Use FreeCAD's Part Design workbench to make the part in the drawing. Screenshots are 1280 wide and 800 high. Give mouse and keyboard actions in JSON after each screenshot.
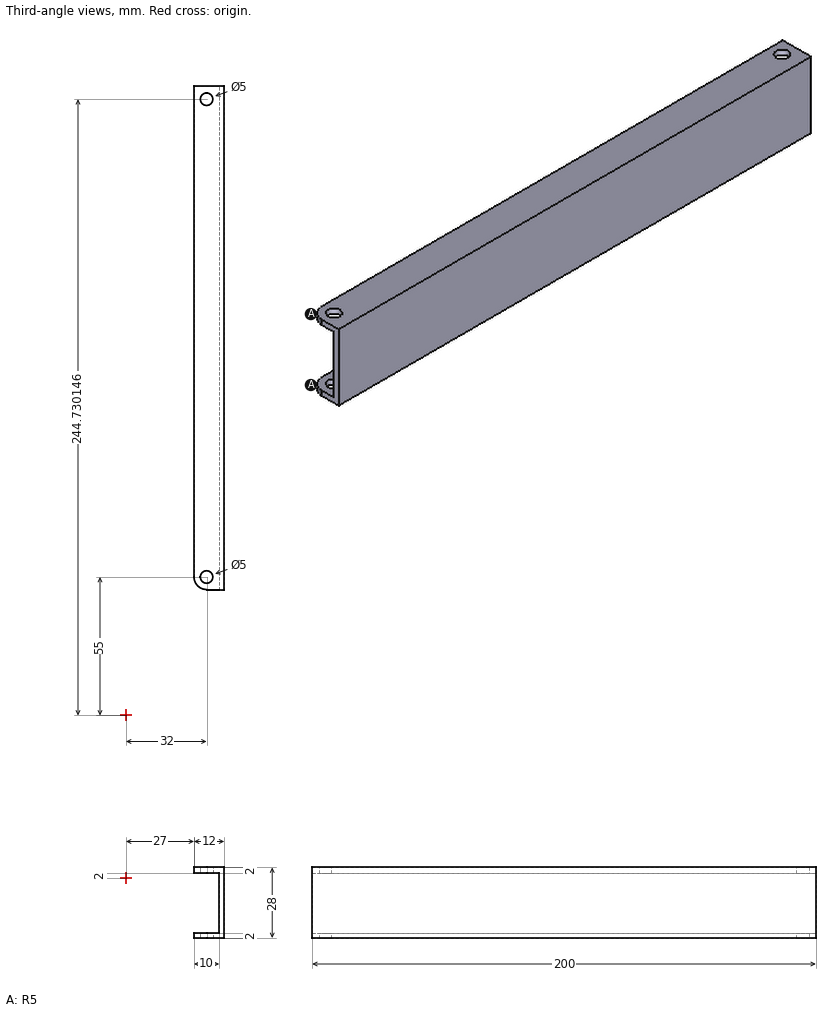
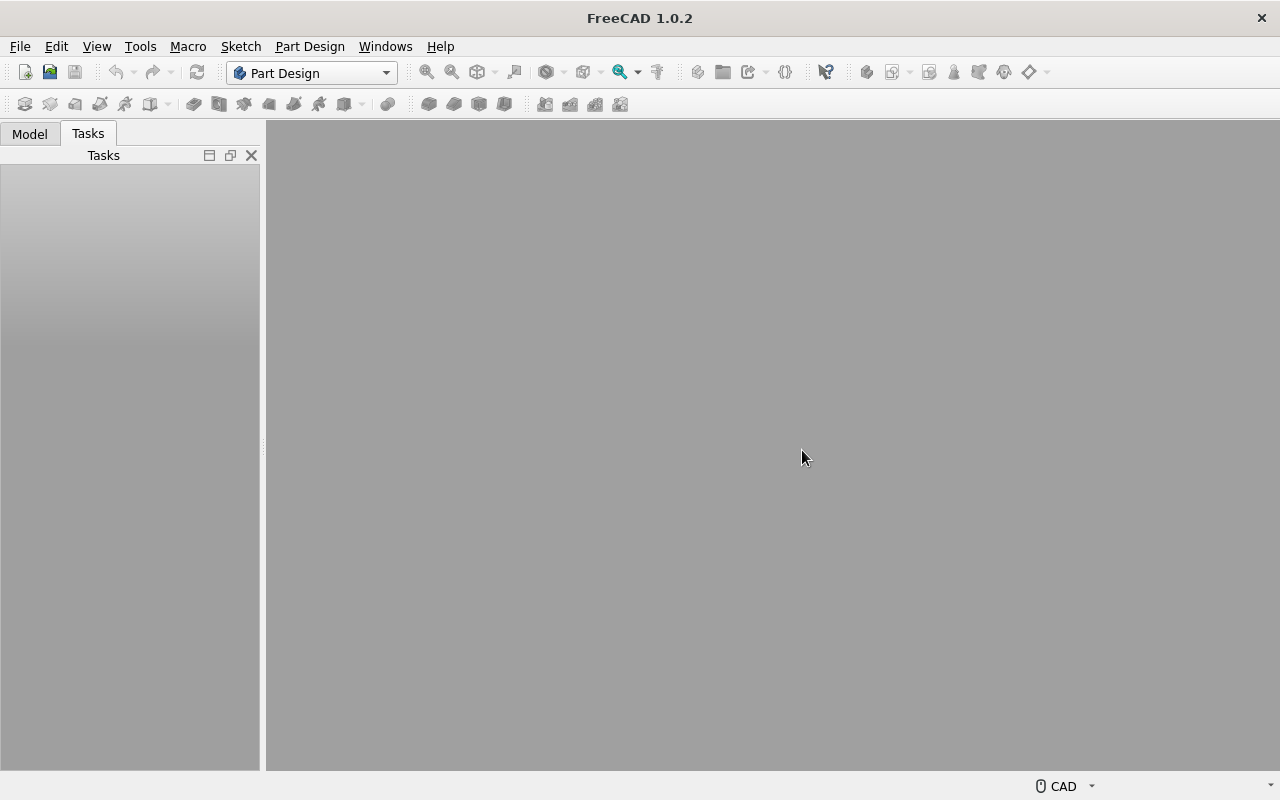
{"action": "left_click", "coordinate": [25, 72]}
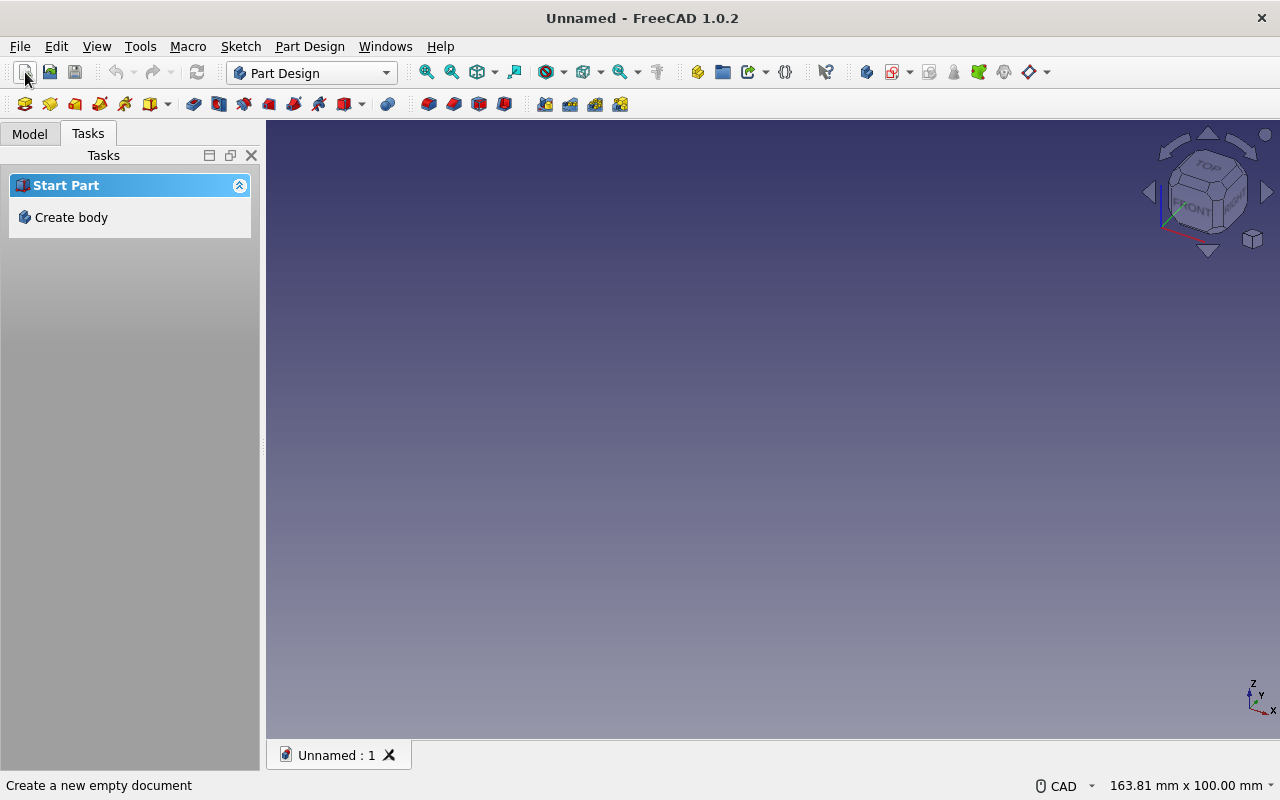
{"action": "left_click", "coordinate": [867, 72]}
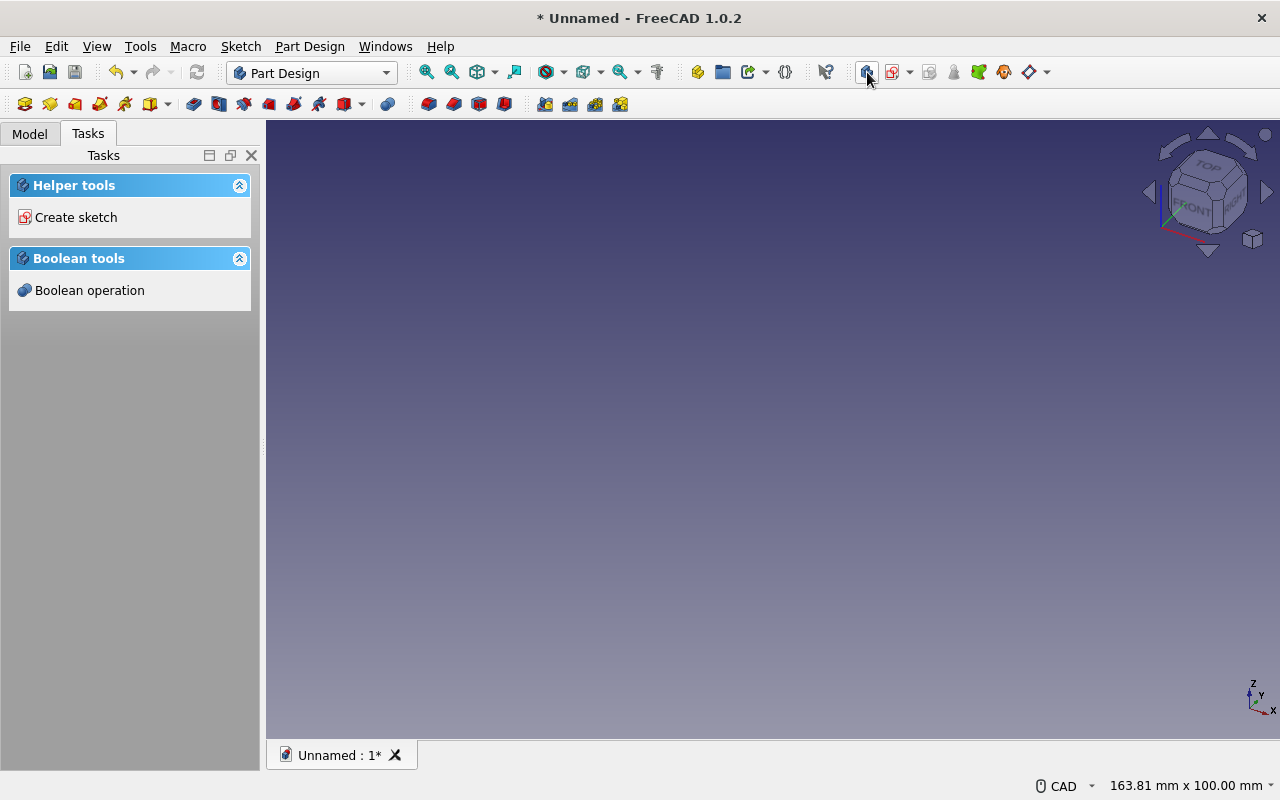
{"action": "left_click", "coordinate": [30, 134]}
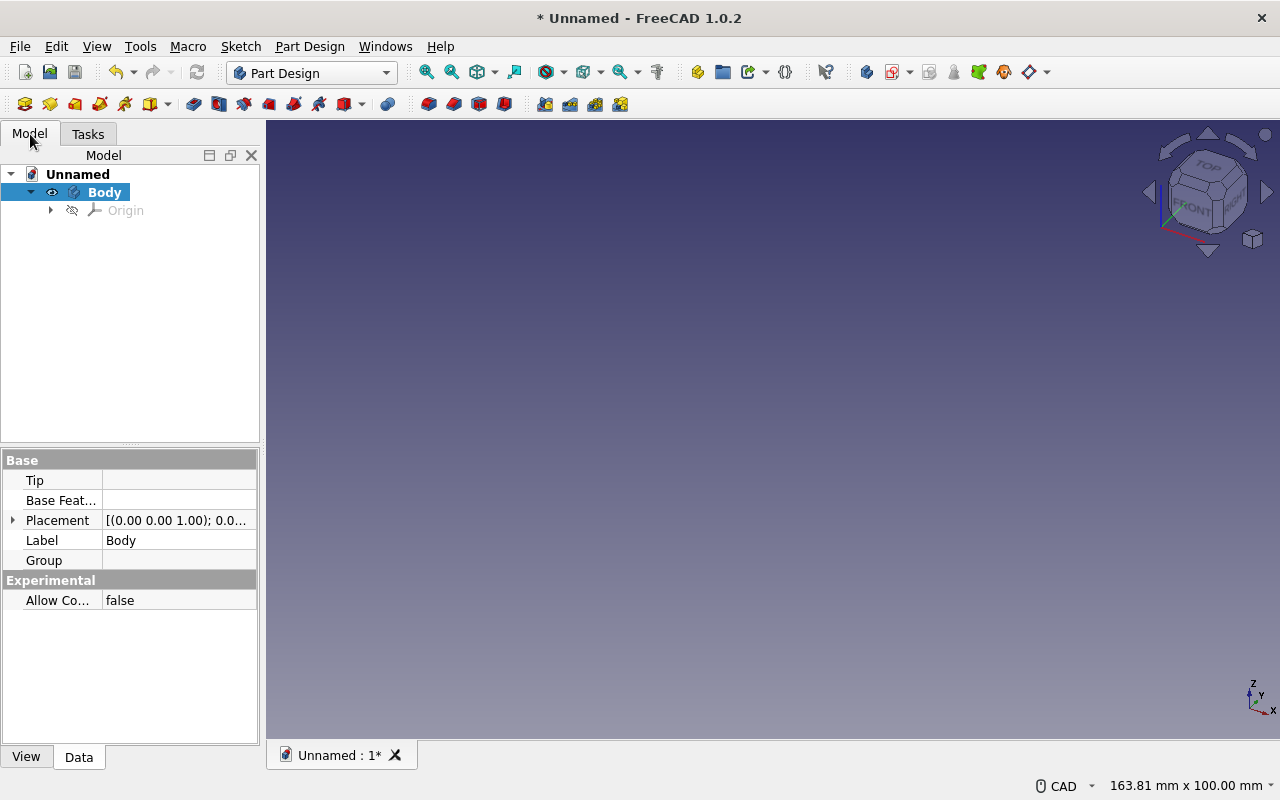
{"action": "left_click", "coordinate": [51, 210]}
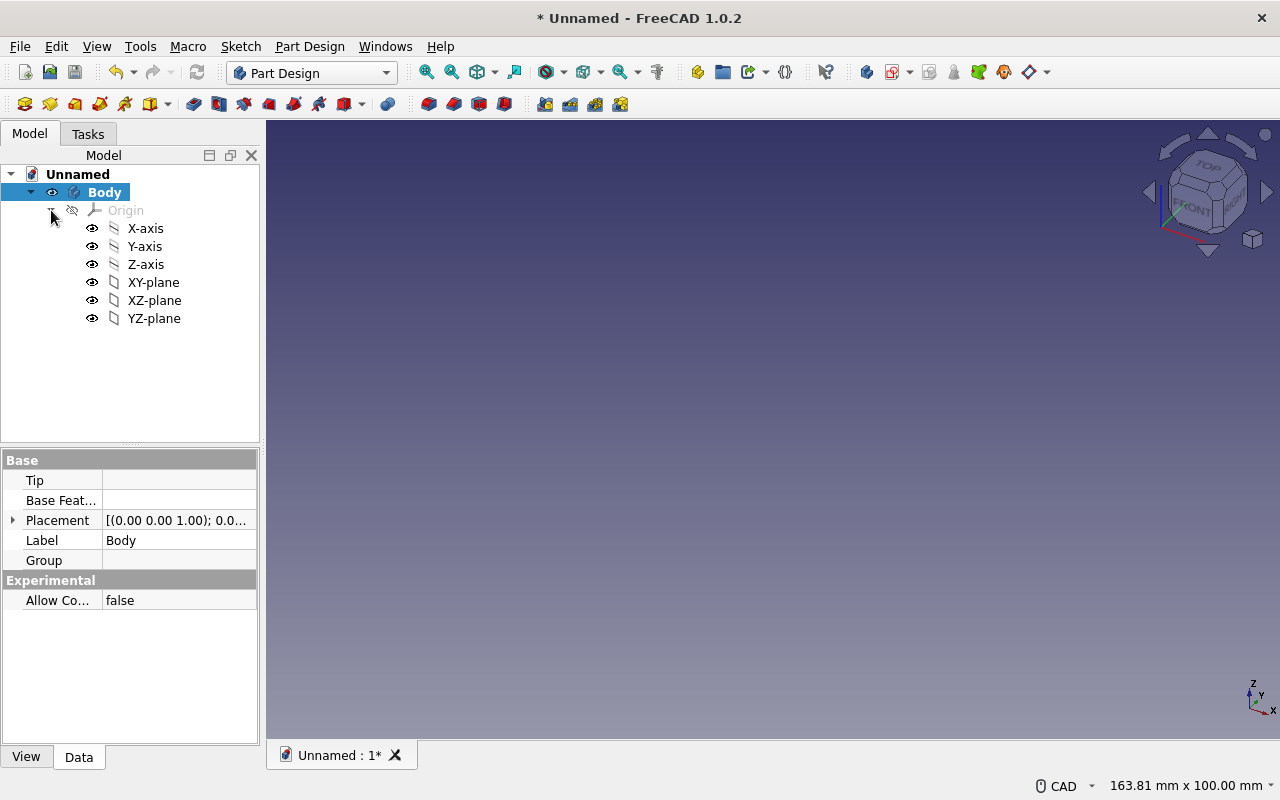
{"action": "left_click", "coordinate": [137, 300]}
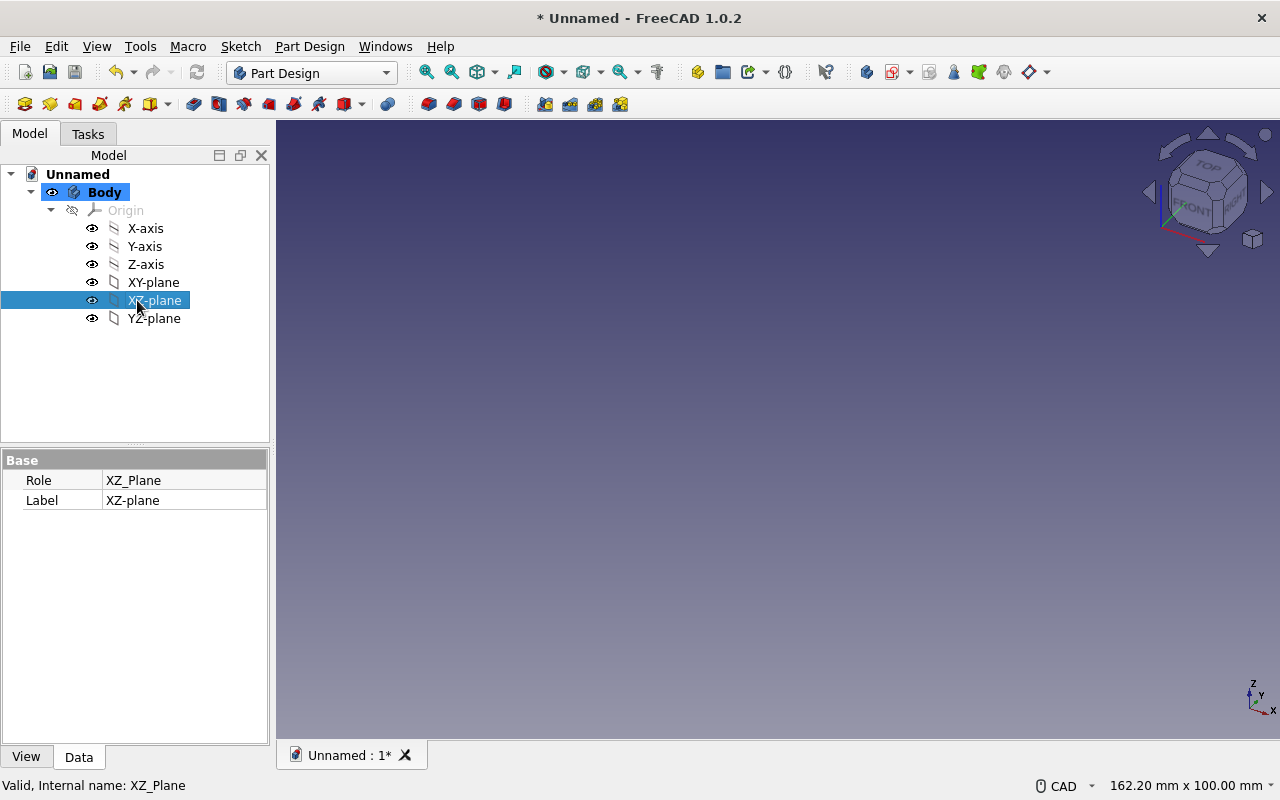
{"action": "left_click", "coordinate": [1028, 72]}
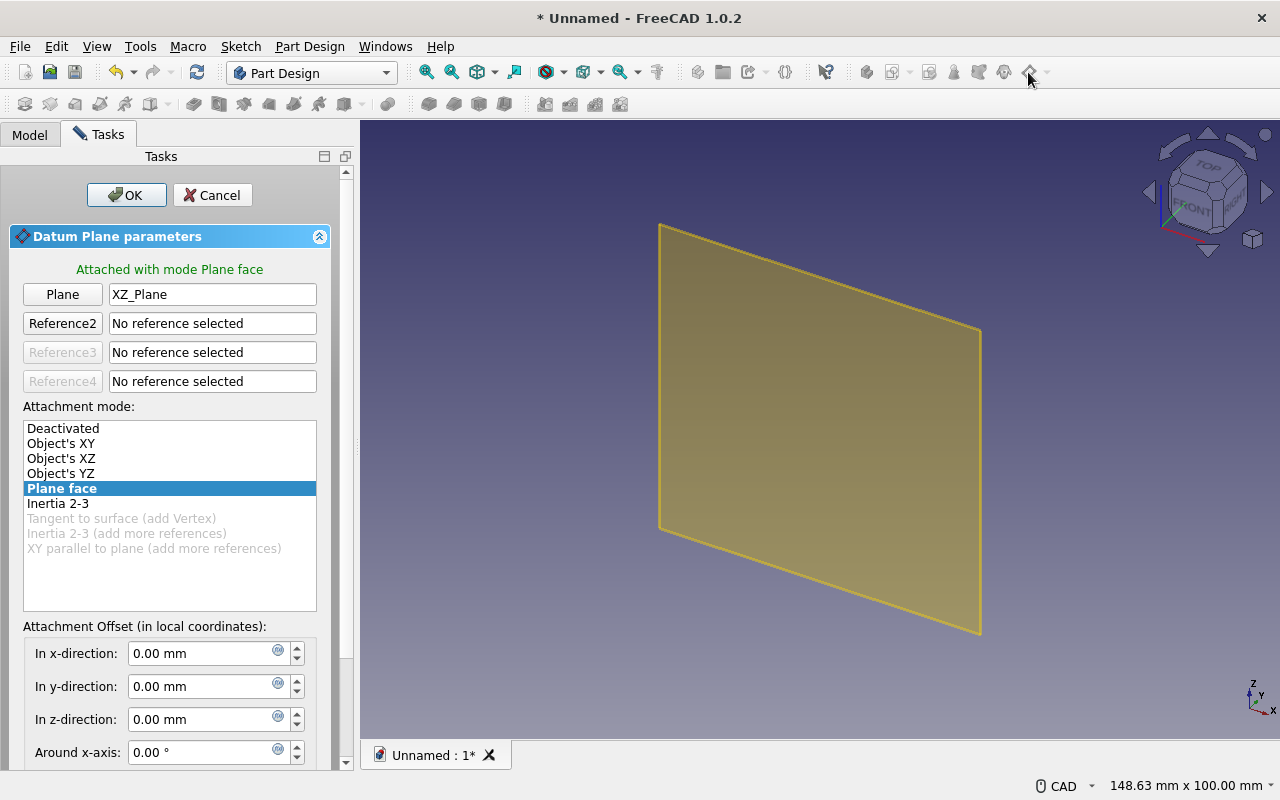
{"action": "triple_click", "coordinate": [210, 720]}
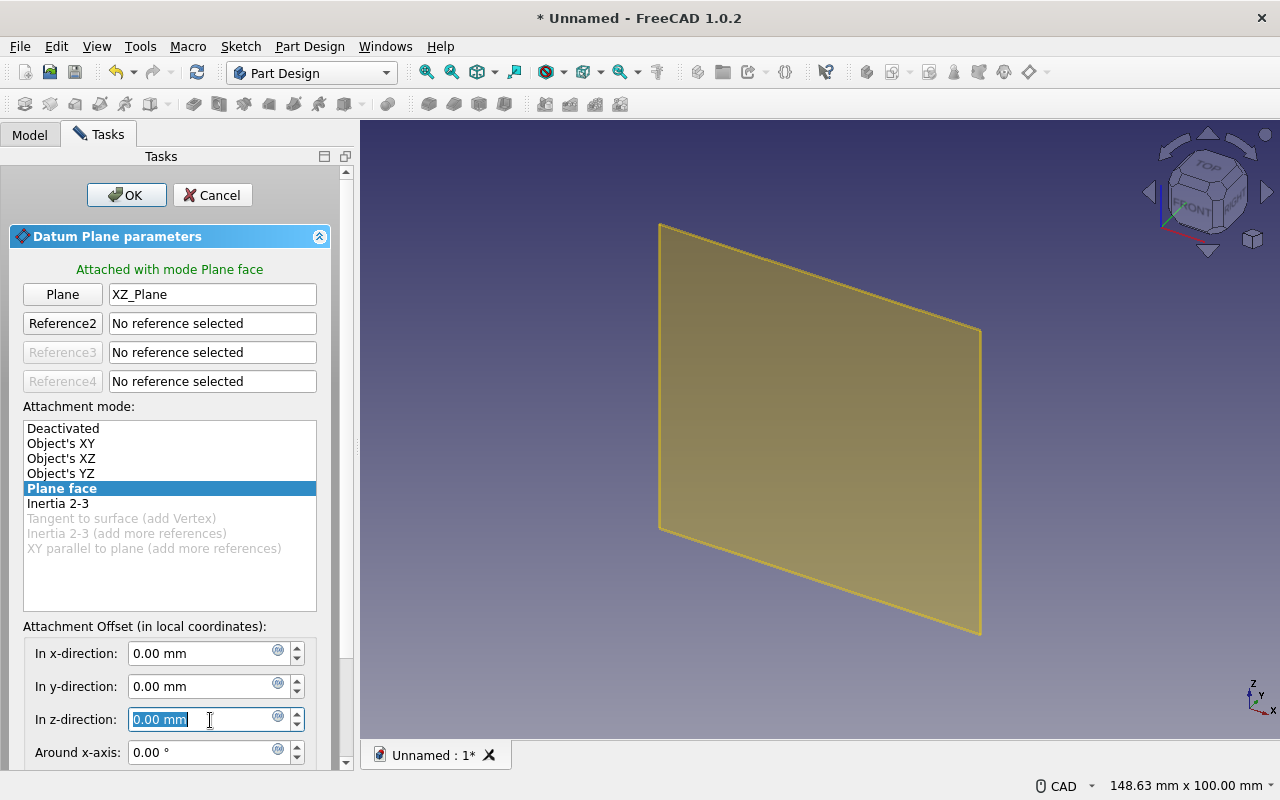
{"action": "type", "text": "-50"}
{"action": "key", "text": "Tab"}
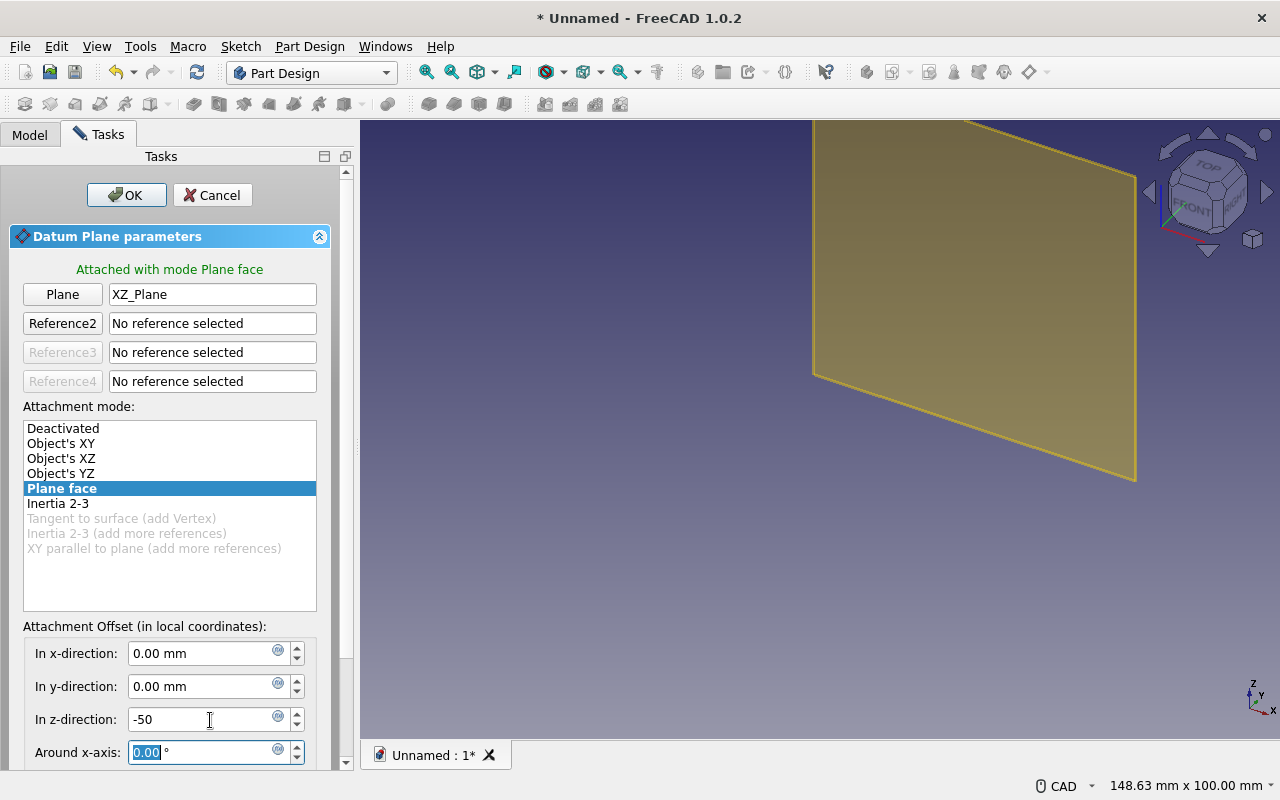
{"action": "left_click", "coordinate": [127, 195]}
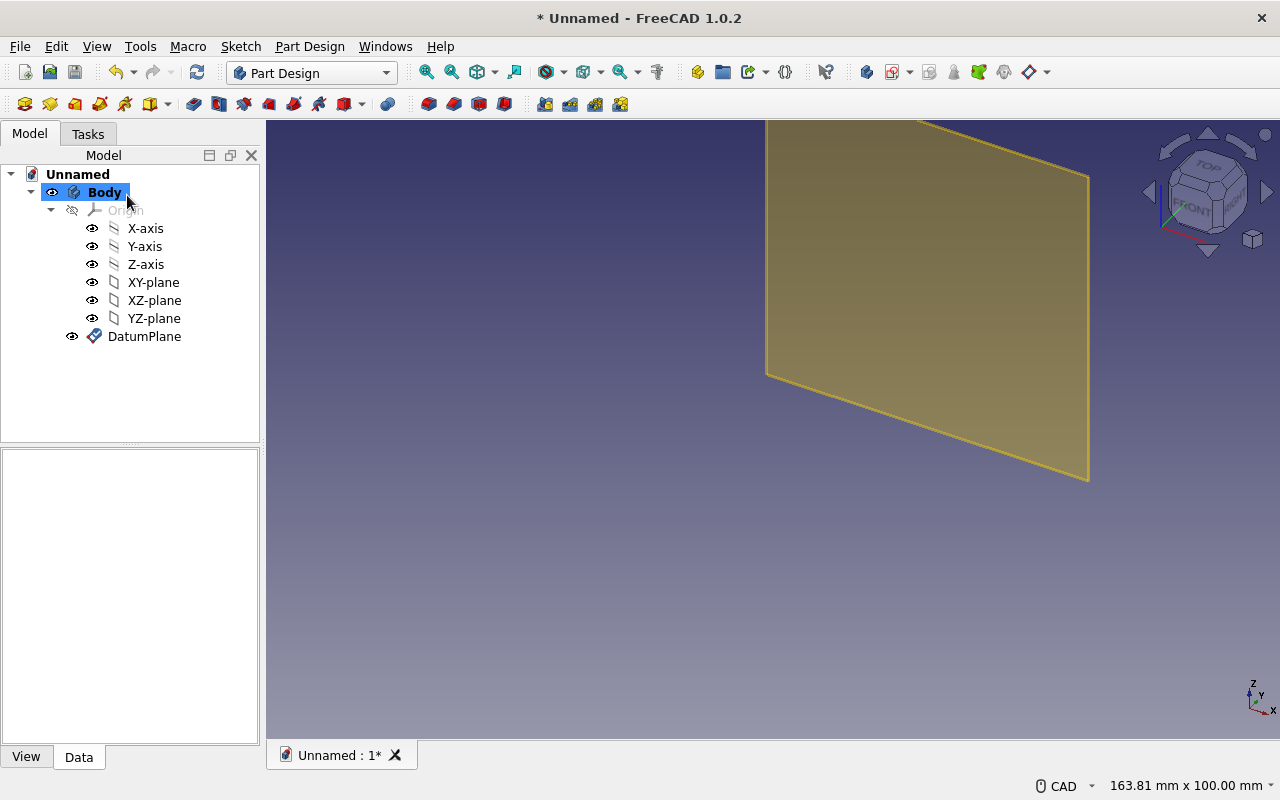
{"action": "left_click", "coordinate": [117, 336]}